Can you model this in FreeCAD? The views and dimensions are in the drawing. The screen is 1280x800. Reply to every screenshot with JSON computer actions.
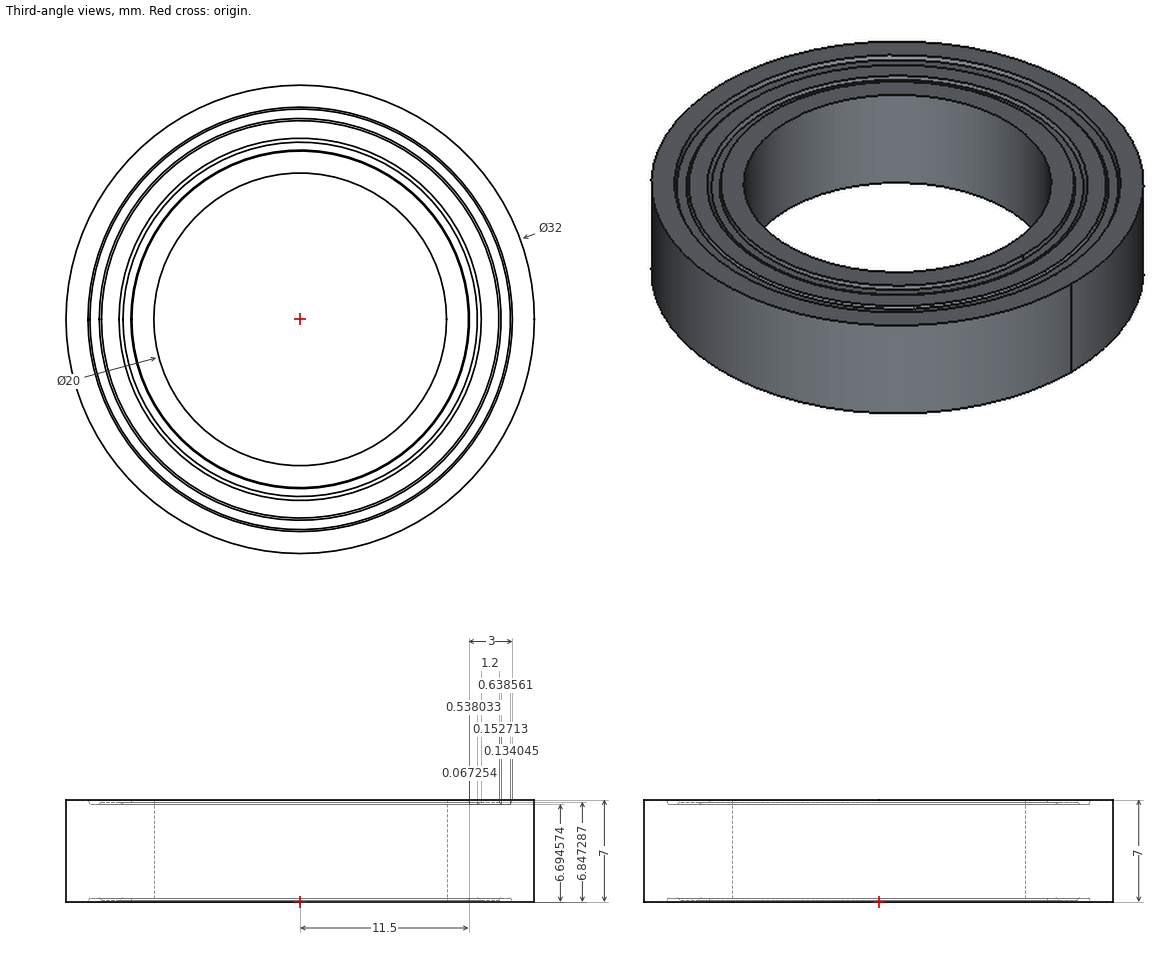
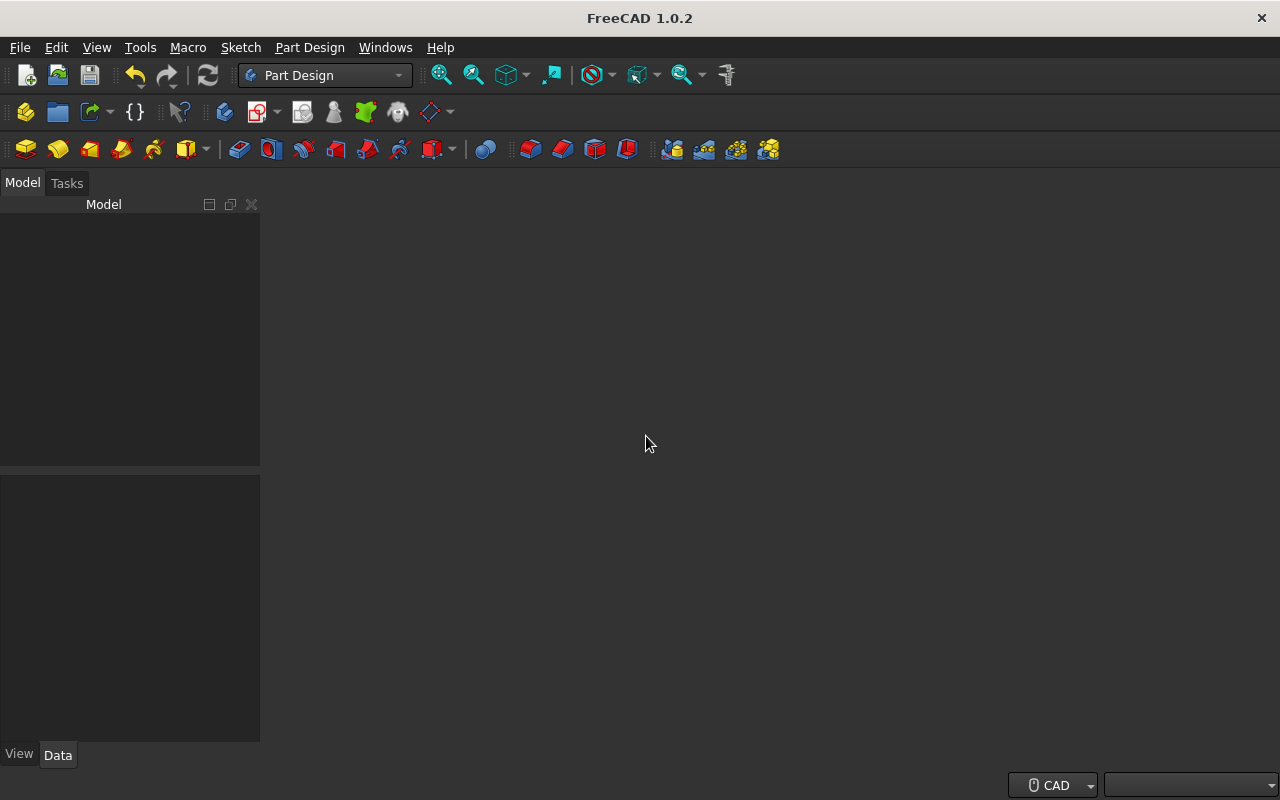
{"action": "key", "text": "ctrl+n"}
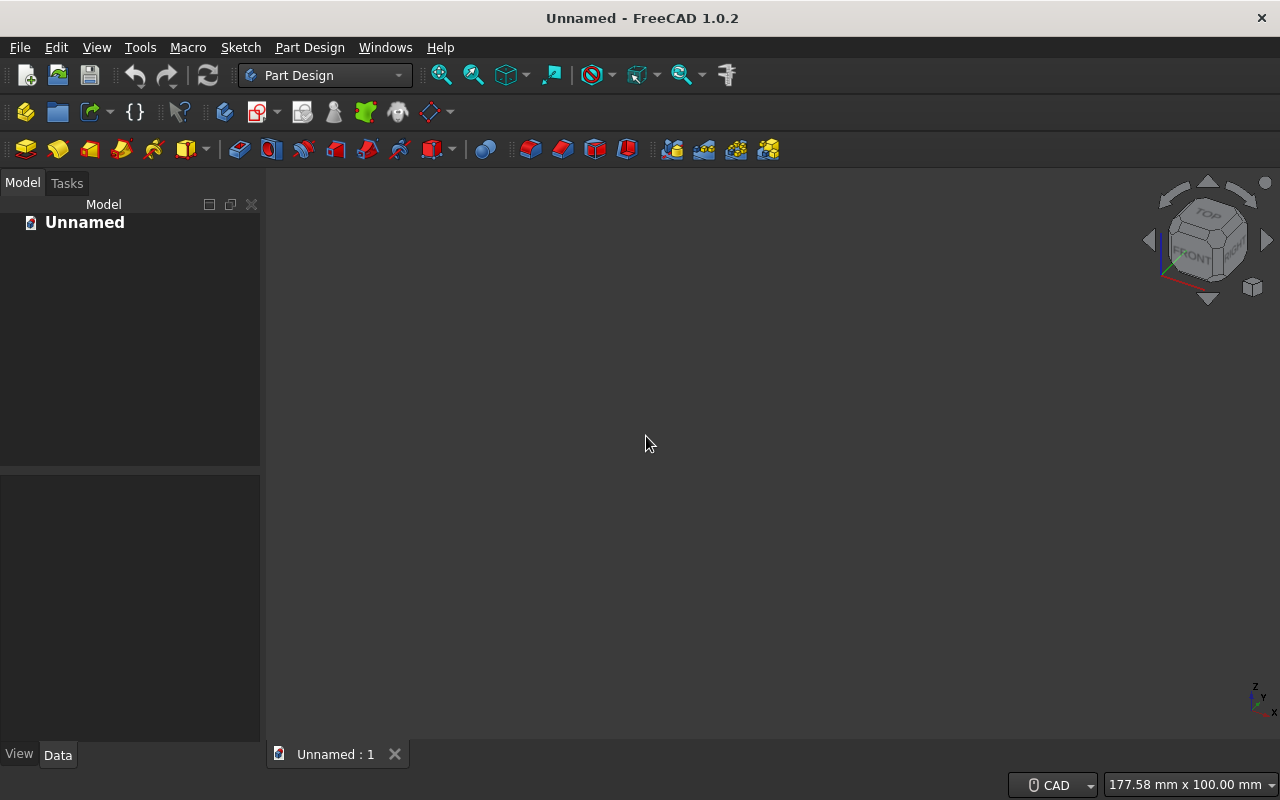
{"action": "left_click", "coordinate": [258, 112]}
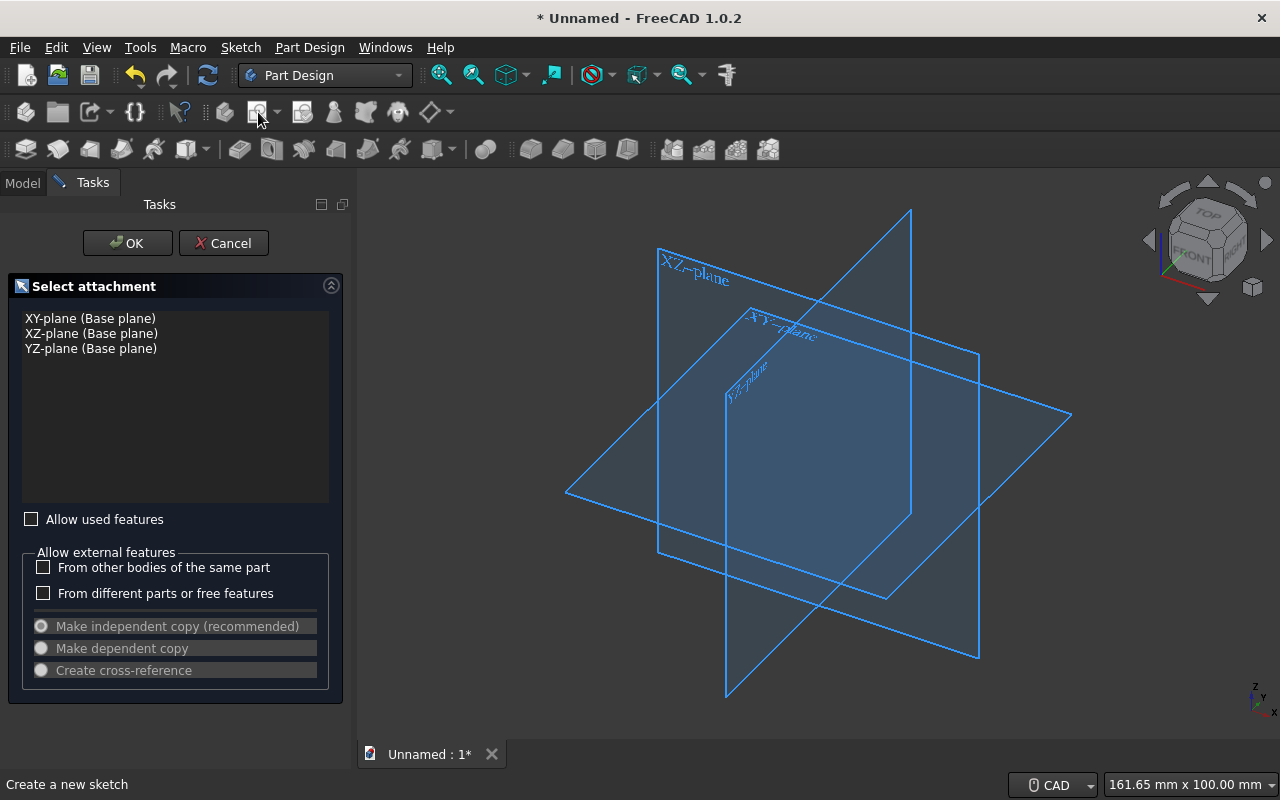
{"action": "left_click", "coordinate": [82, 318]}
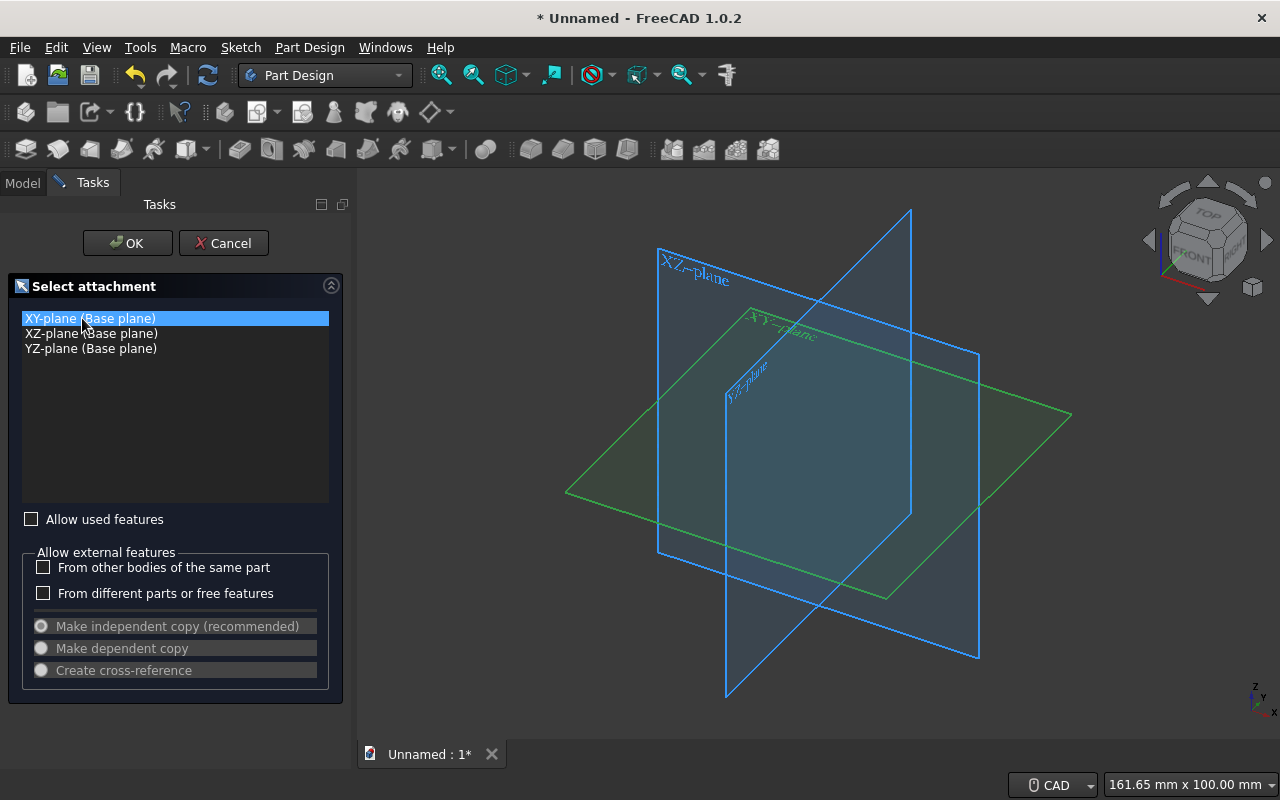
{"action": "left_click", "coordinate": [128, 243]}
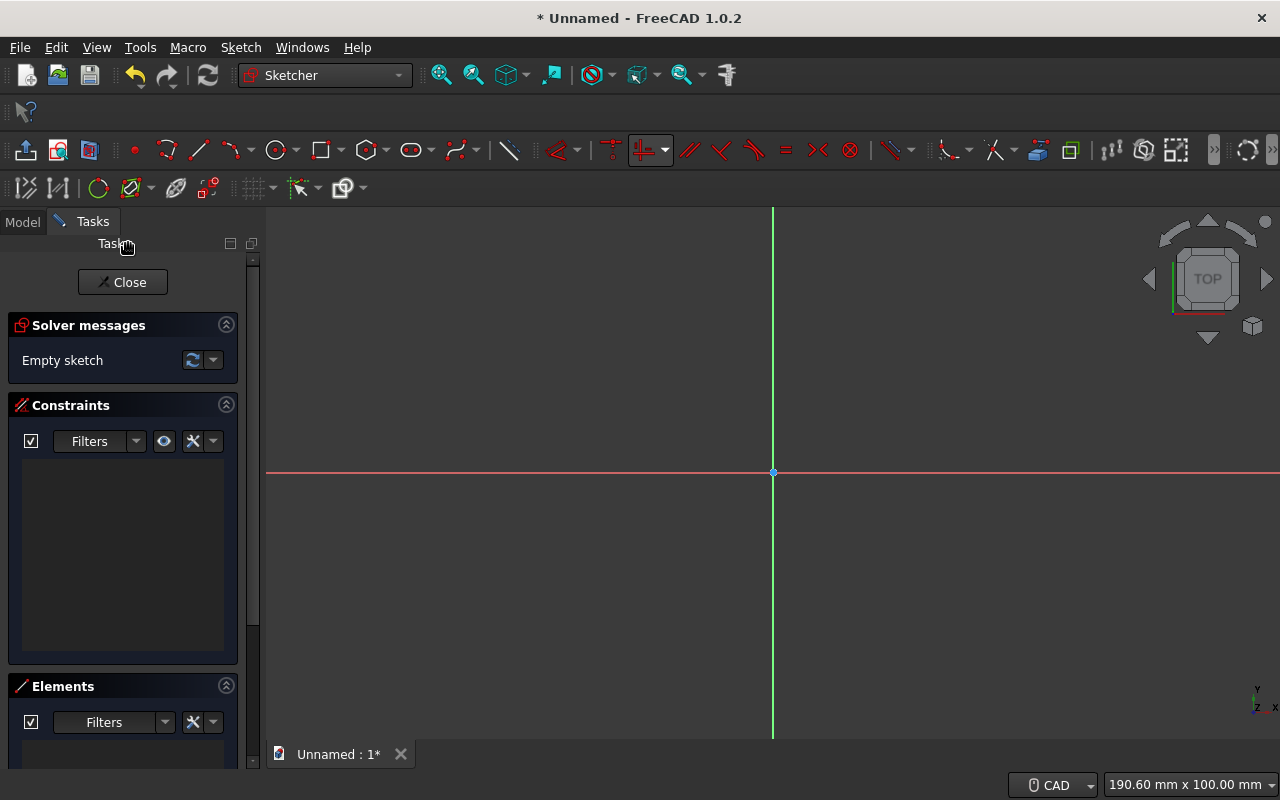
{"action": "scroll", "coordinate": [856, 473], "scroll_direction": "up", "scroll_amount": 3}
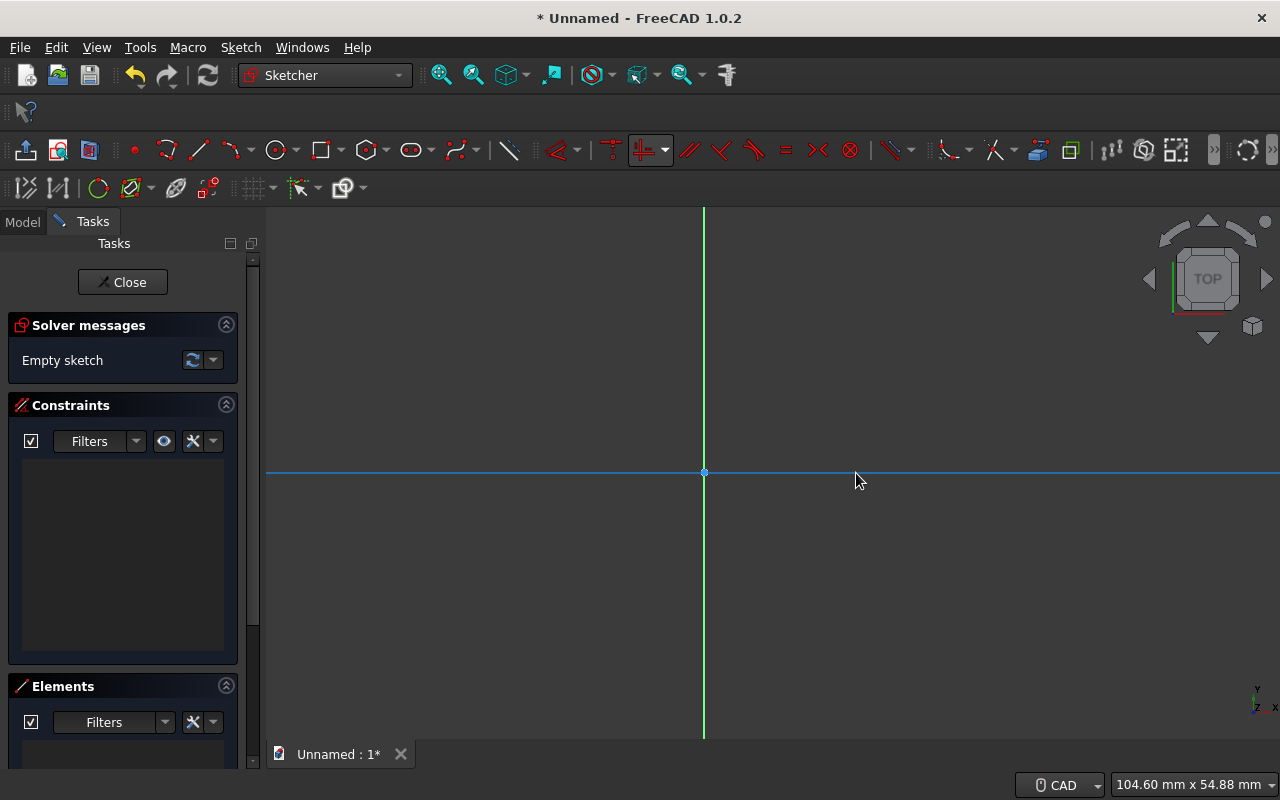
{"action": "left_click", "coordinate": [276, 150]}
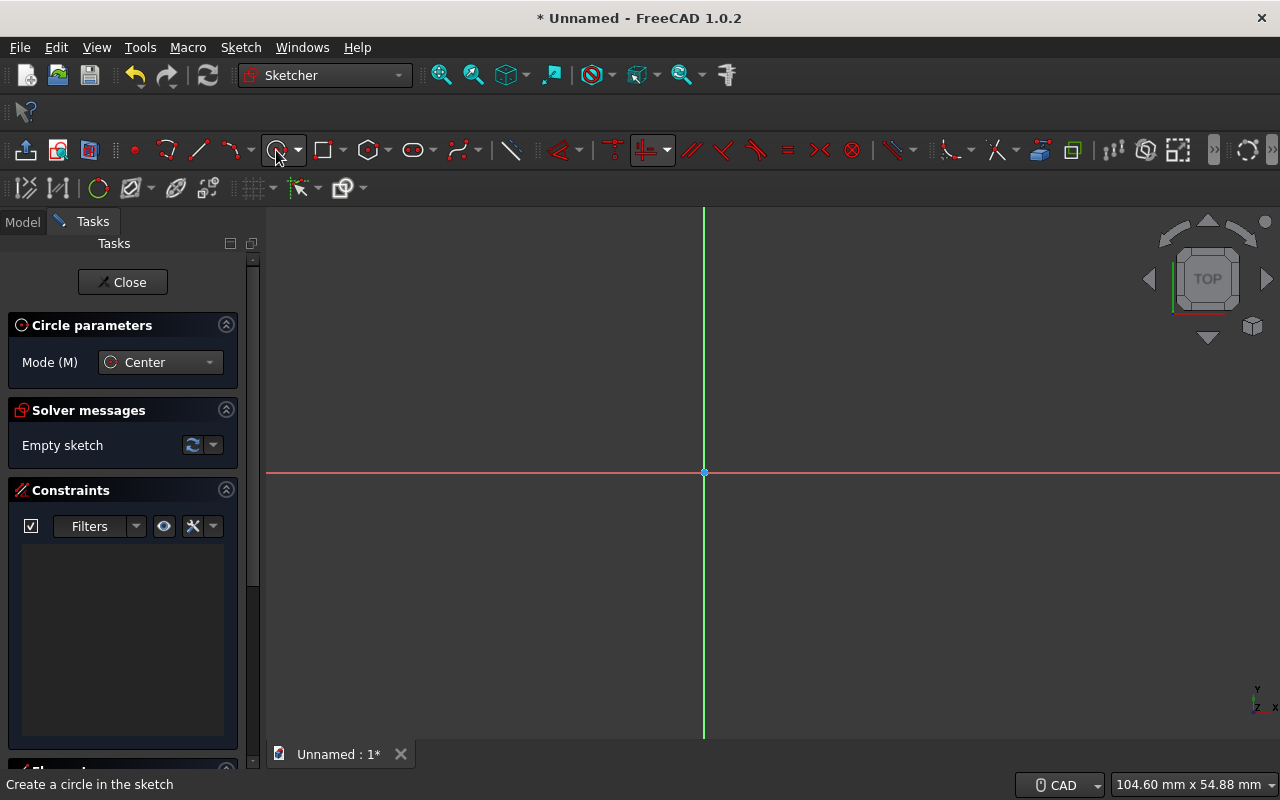
{"action": "left_click", "coordinate": [704, 473]}
{"action": "left_click", "coordinate": [814, 363]}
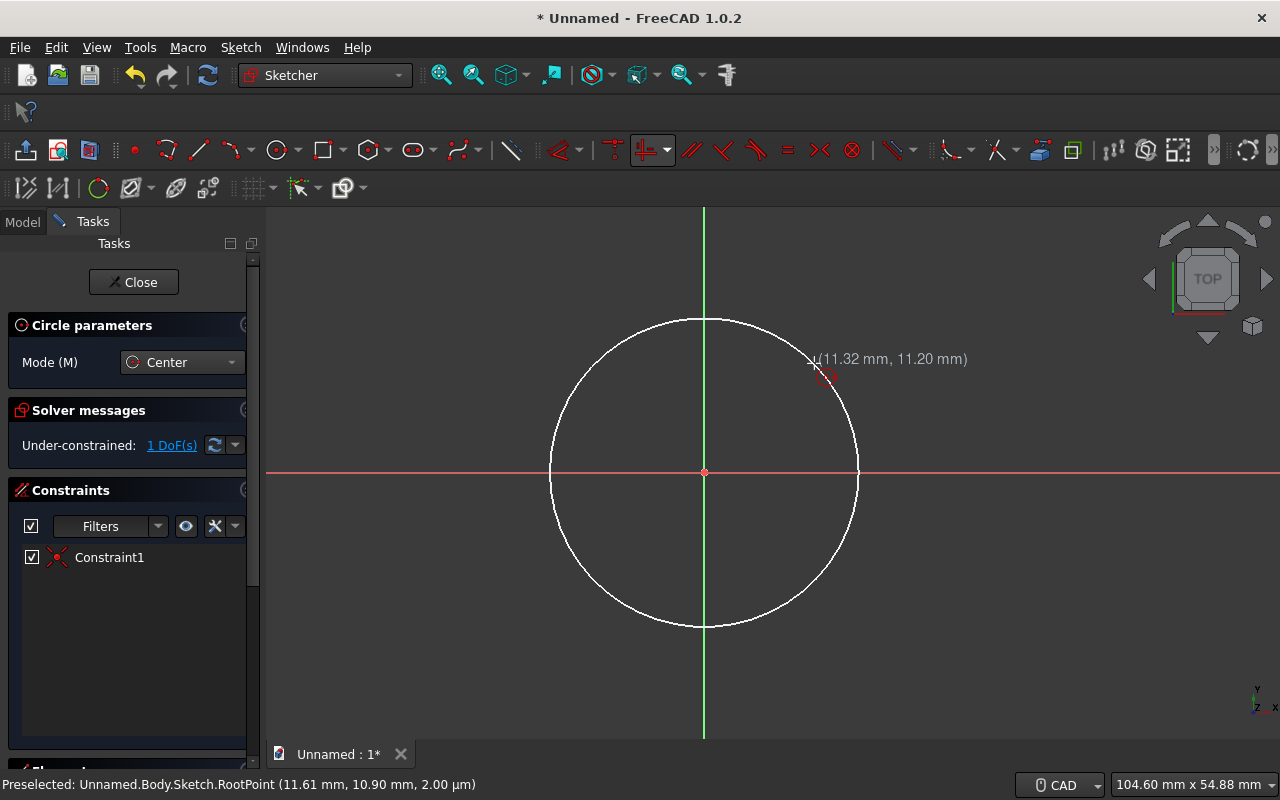
{"action": "left_click", "coordinate": [704, 473]}
{"action": "left_click", "coordinate": [773, 404]}
{"action": "key", "text": "Escape"}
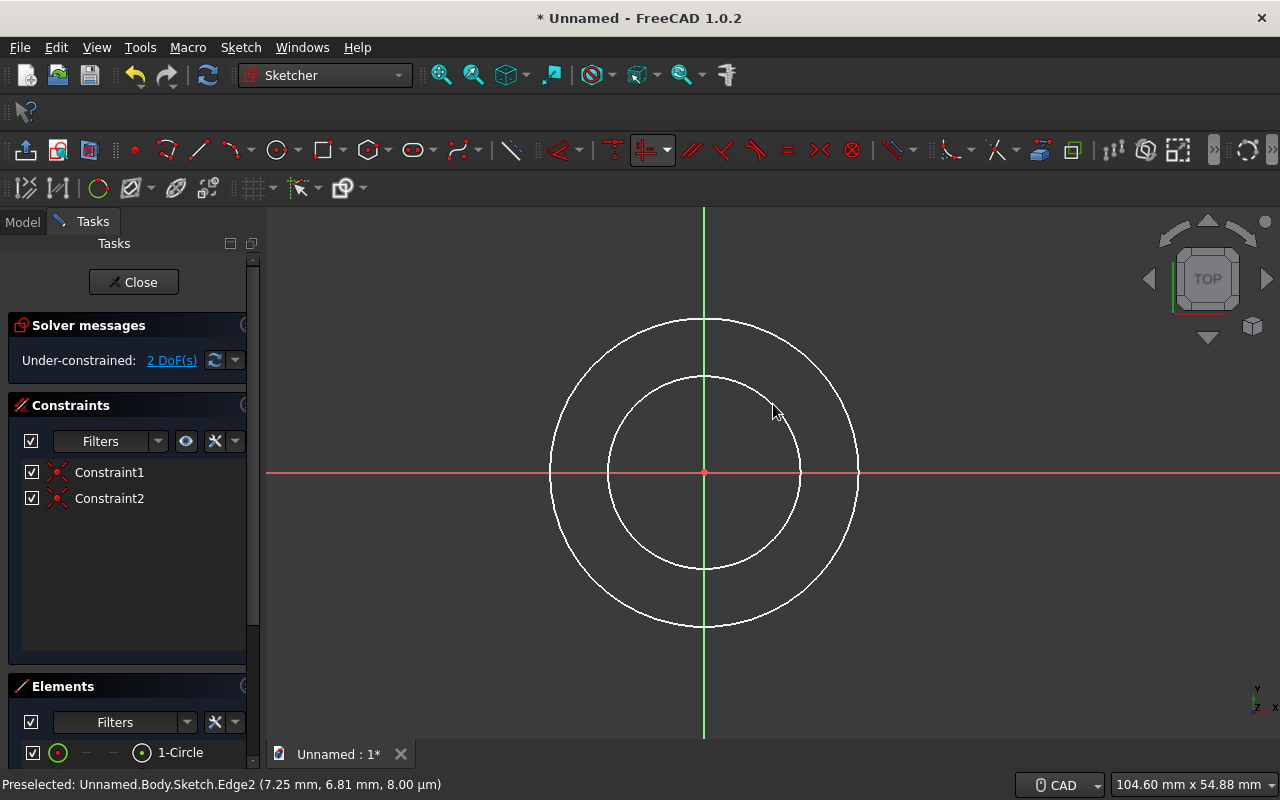
{"action": "key", "text": "d"}